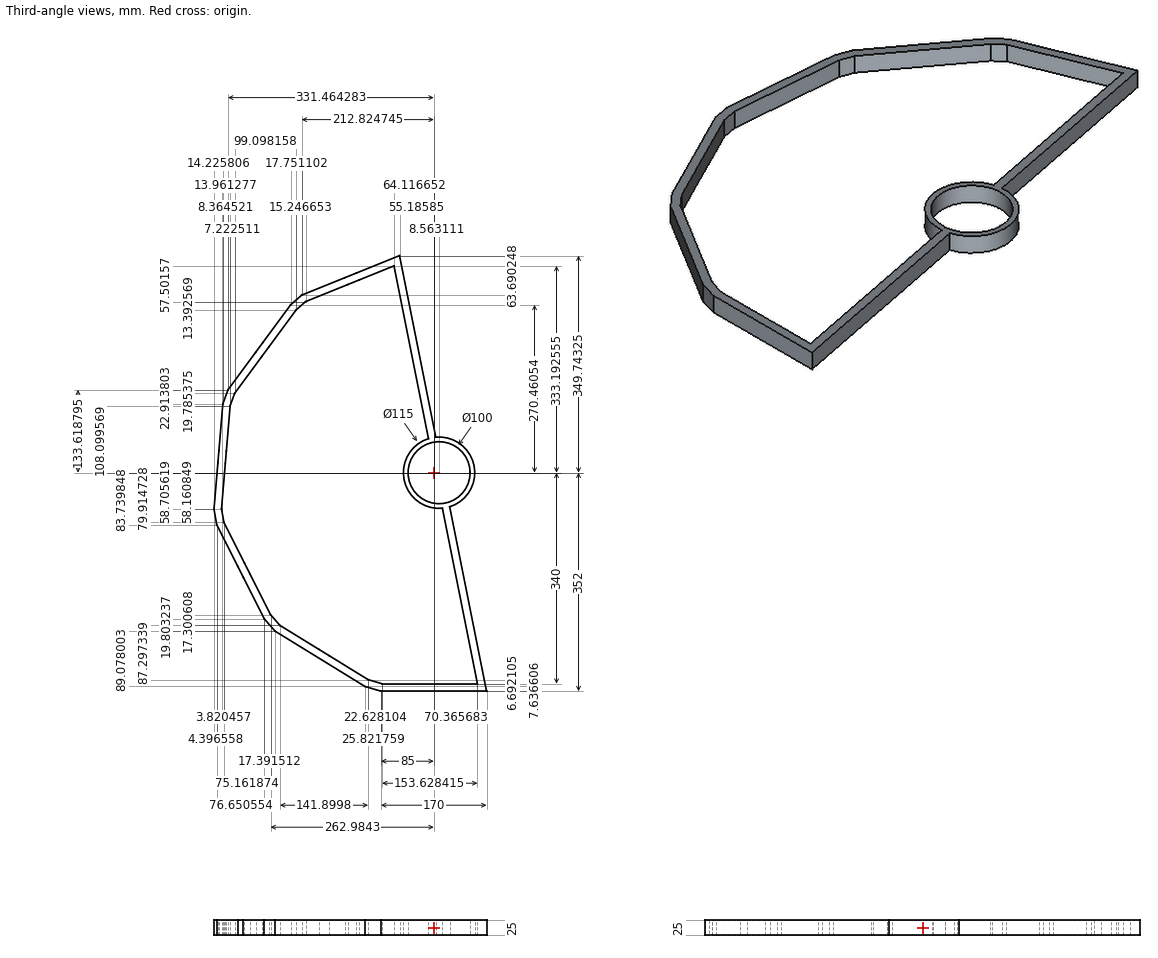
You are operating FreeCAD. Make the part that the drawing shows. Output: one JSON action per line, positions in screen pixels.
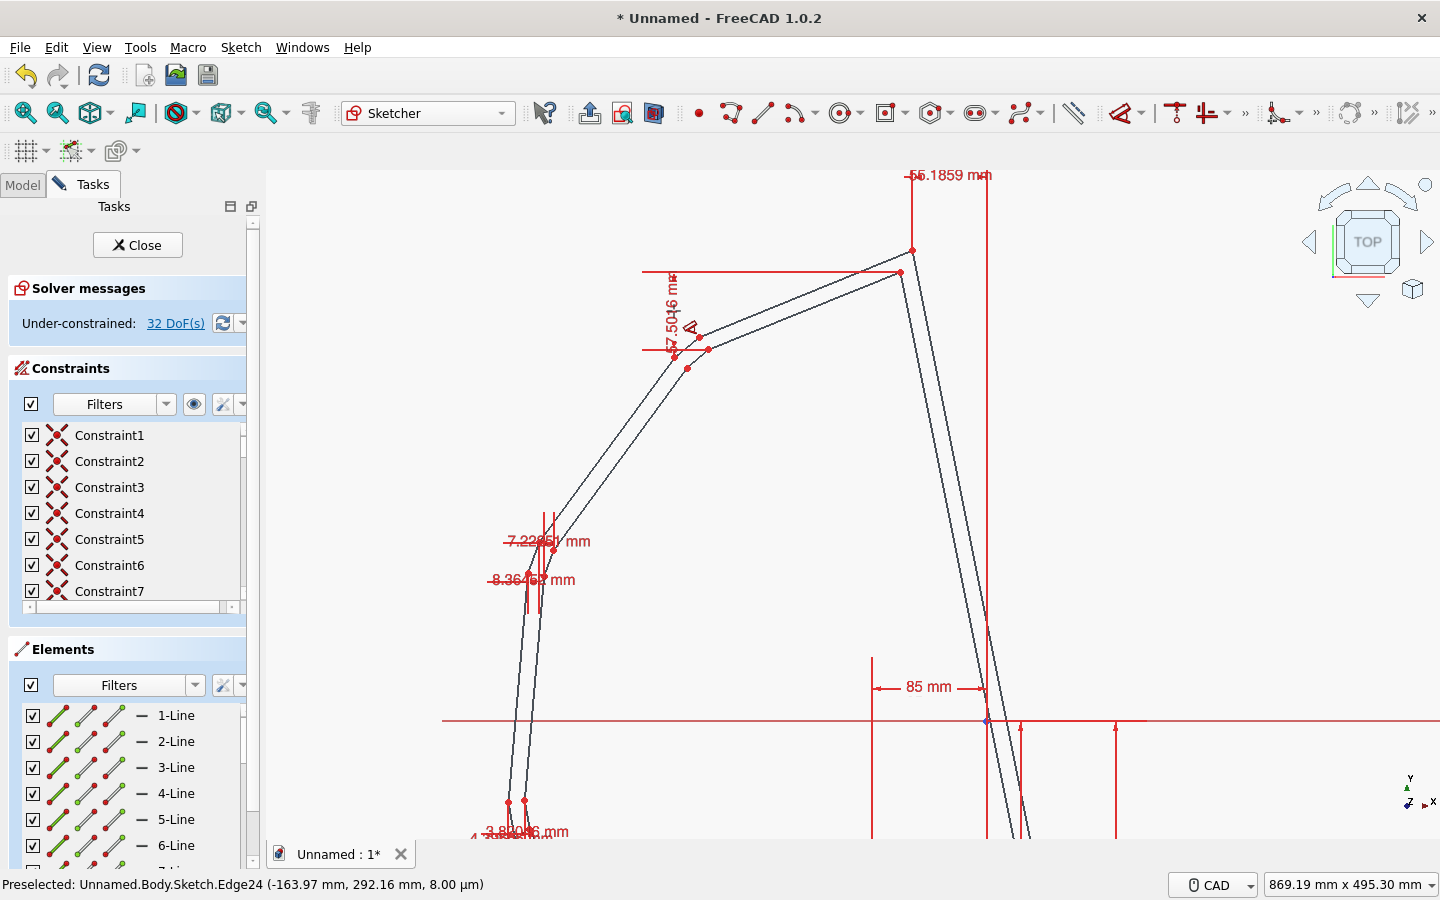
{"action": "scroll", "coordinate": [768, 326], "scroll_direction": "down", "scroll_amount": 4}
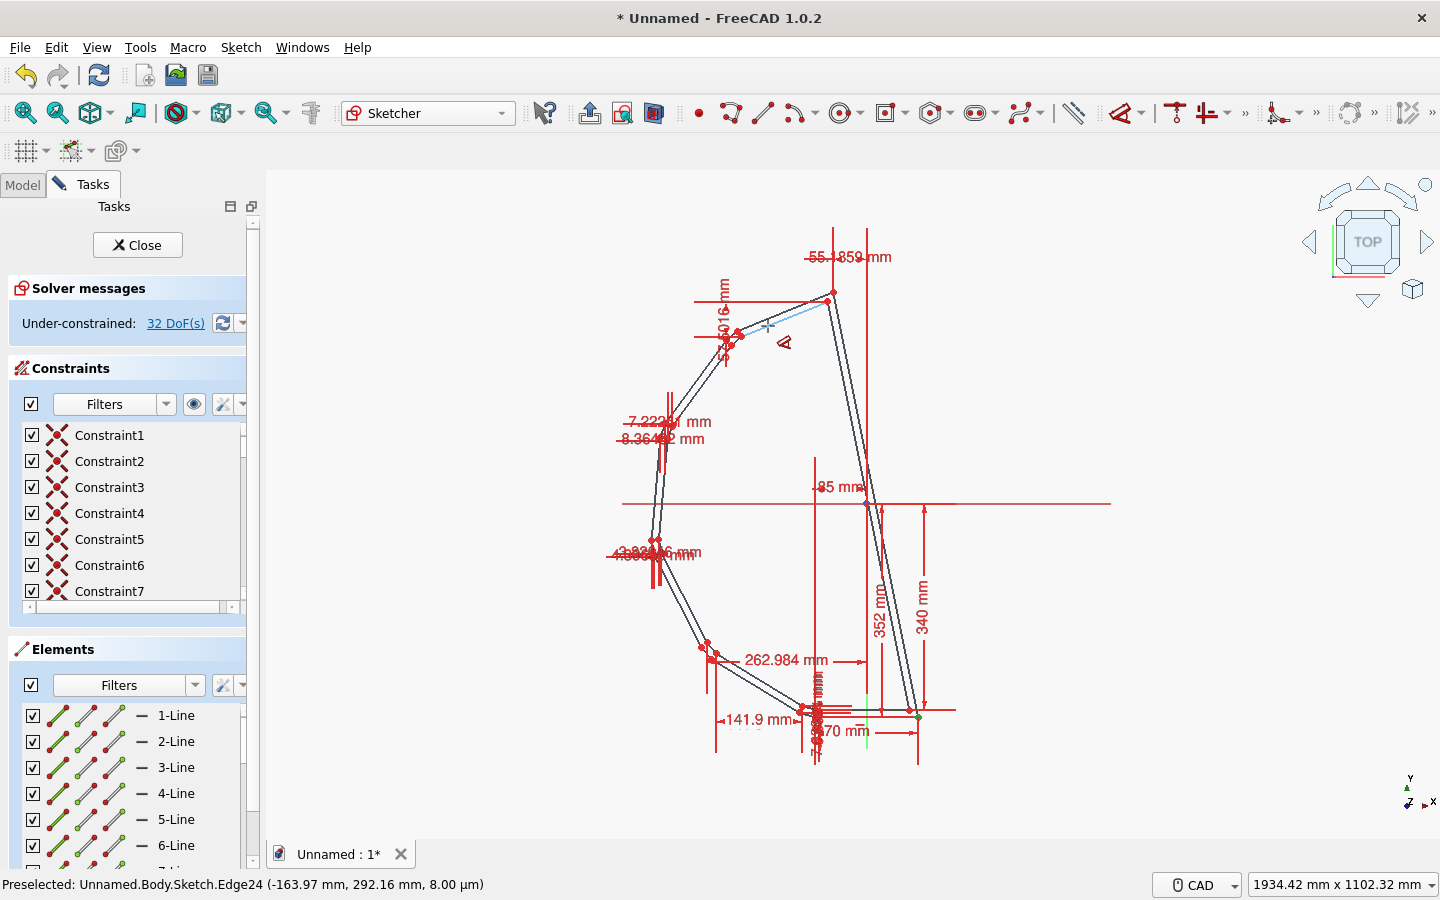
{"action": "scroll", "coordinate": [881, 710], "scroll_direction": "up", "scroll_amount": 4}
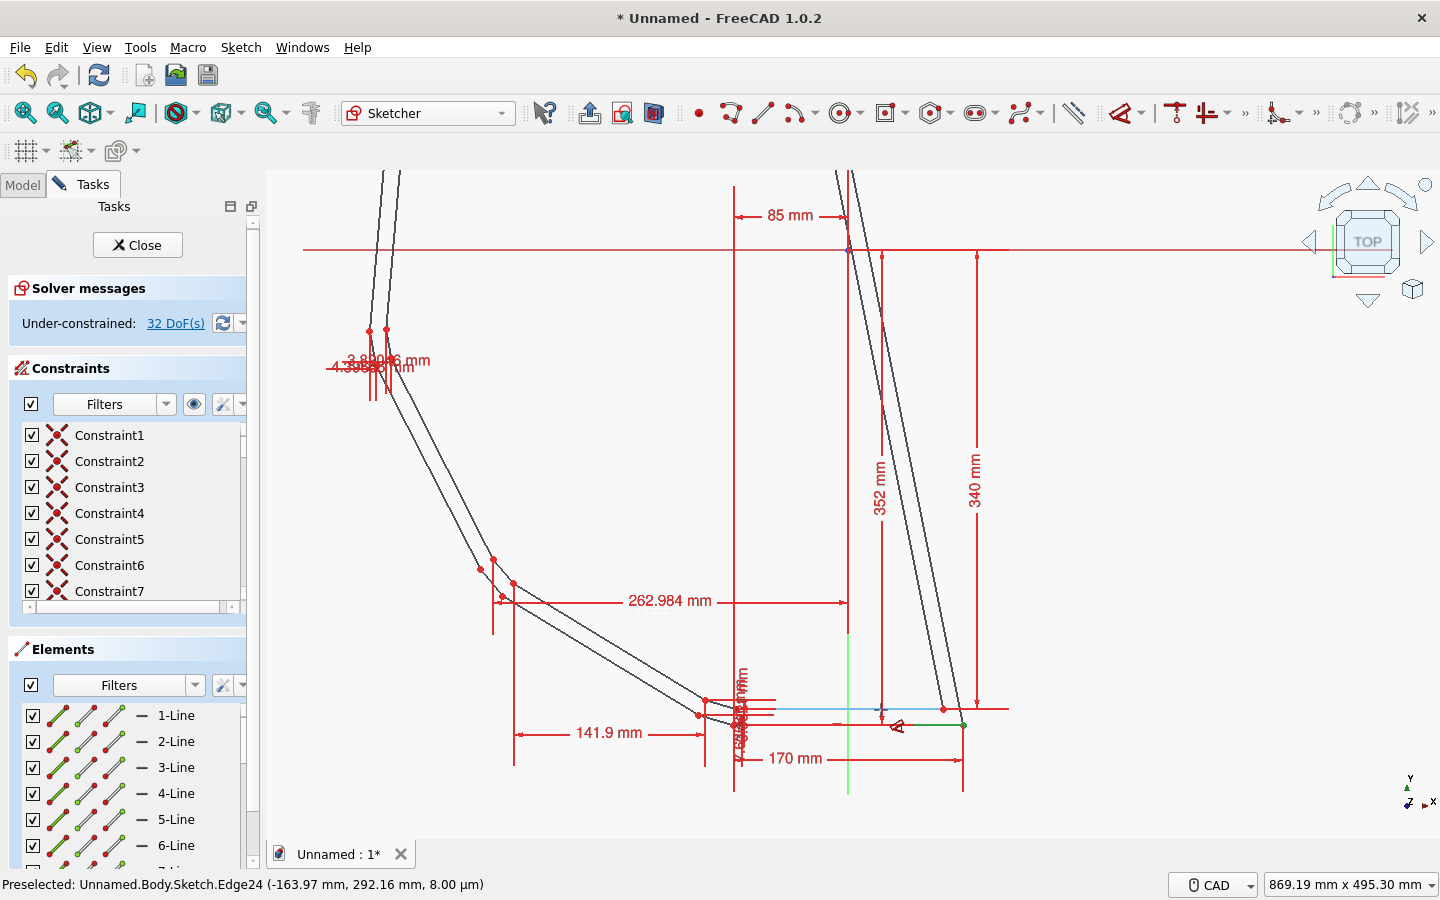
{"action": "left_click", "coordinate": [881, 709]}
{"action": "left_click", "coordinate": [887, 743]}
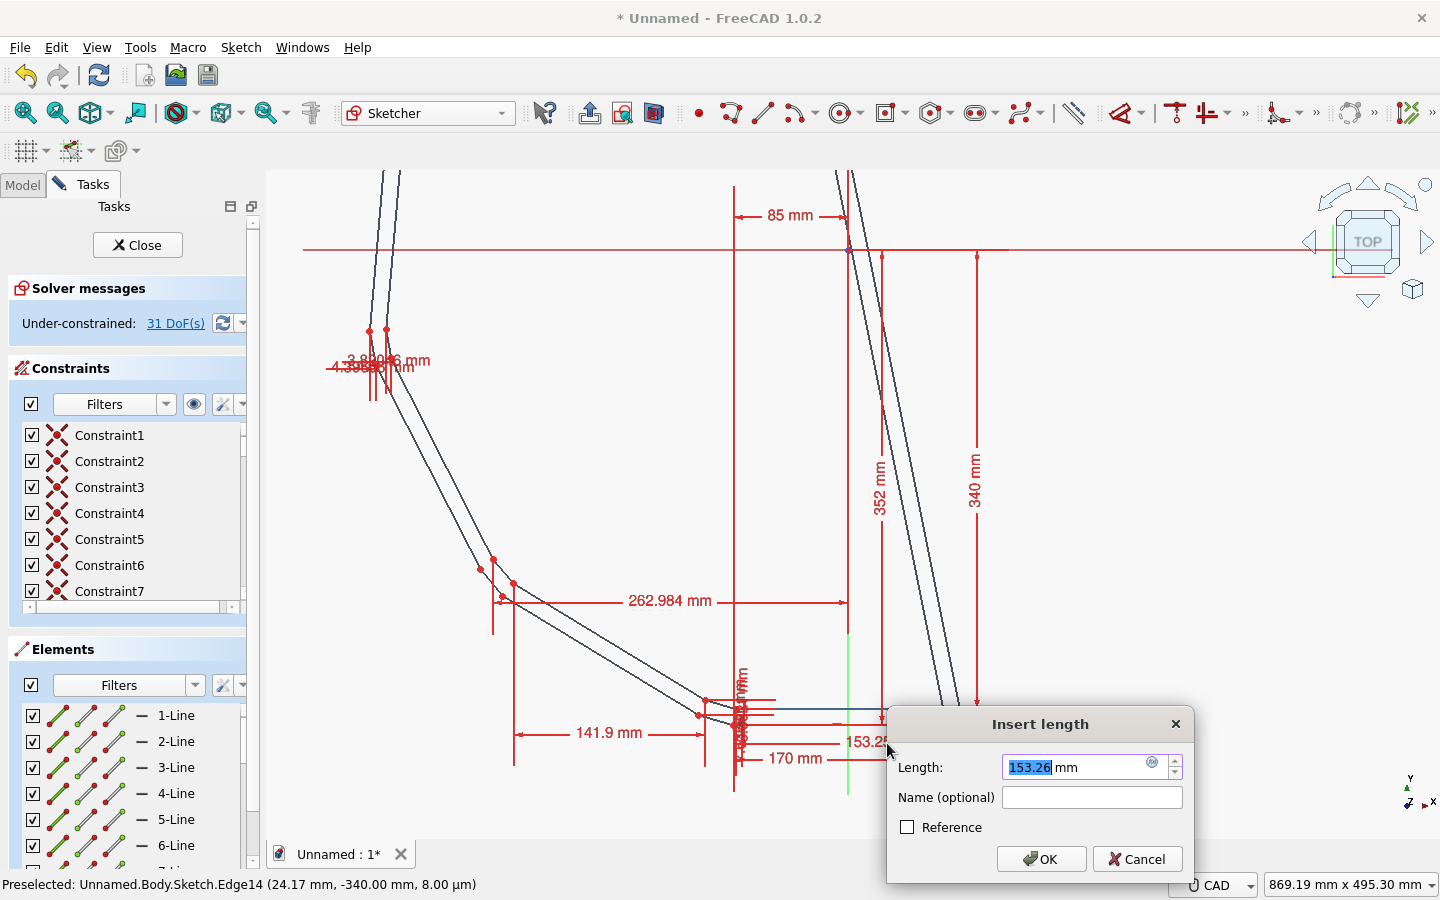
{"action": "type", "text": "153.628415"}
{"action": "key", "text": "Return"}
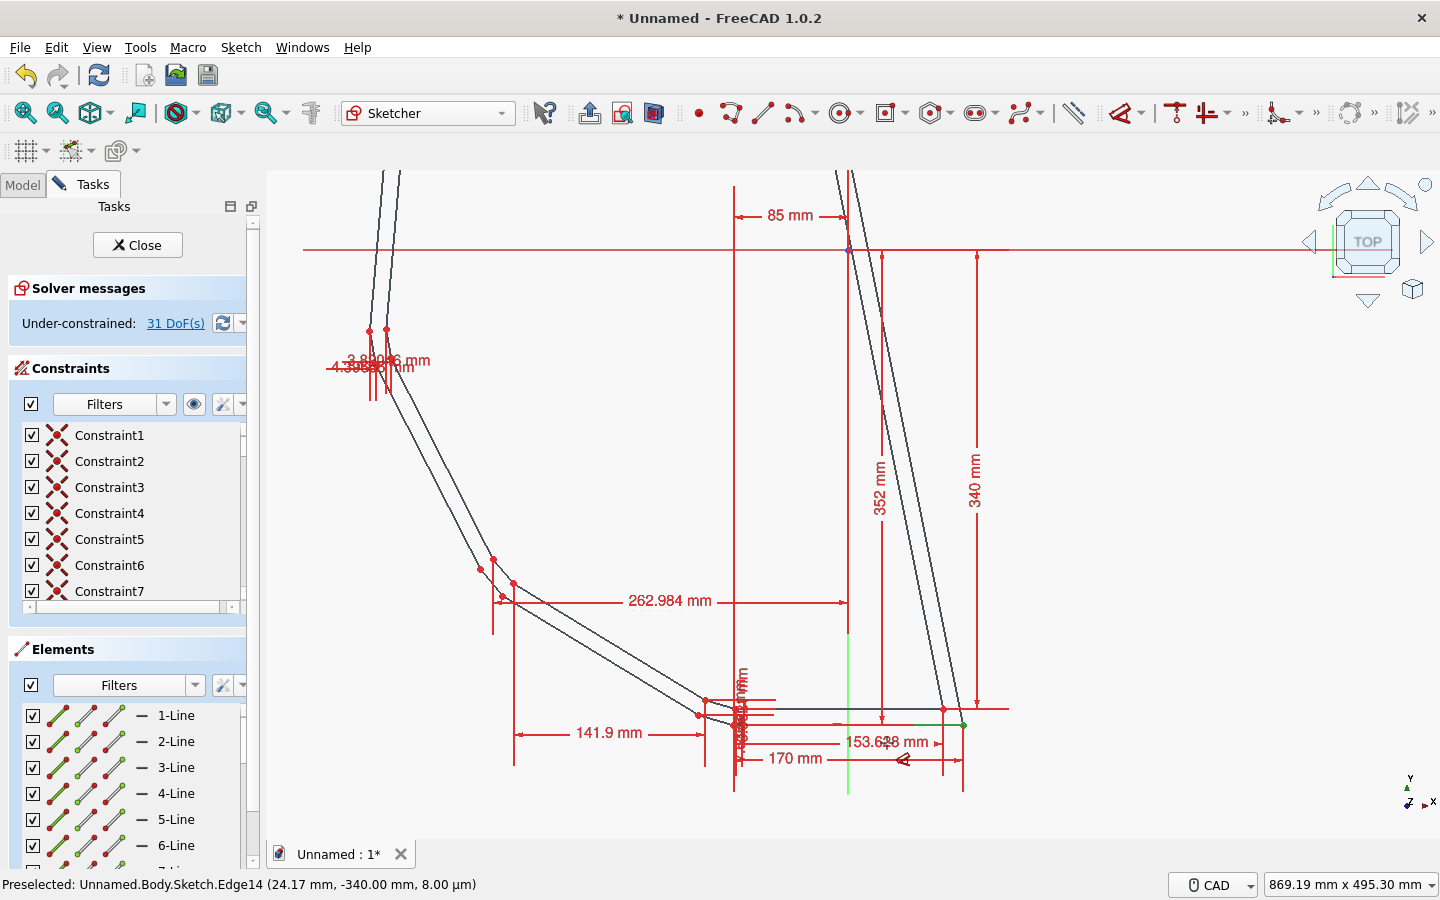
{"action": "scroll", "coordinate": [881, 711], "scroll_direction": "down", "scroll_amount": 4}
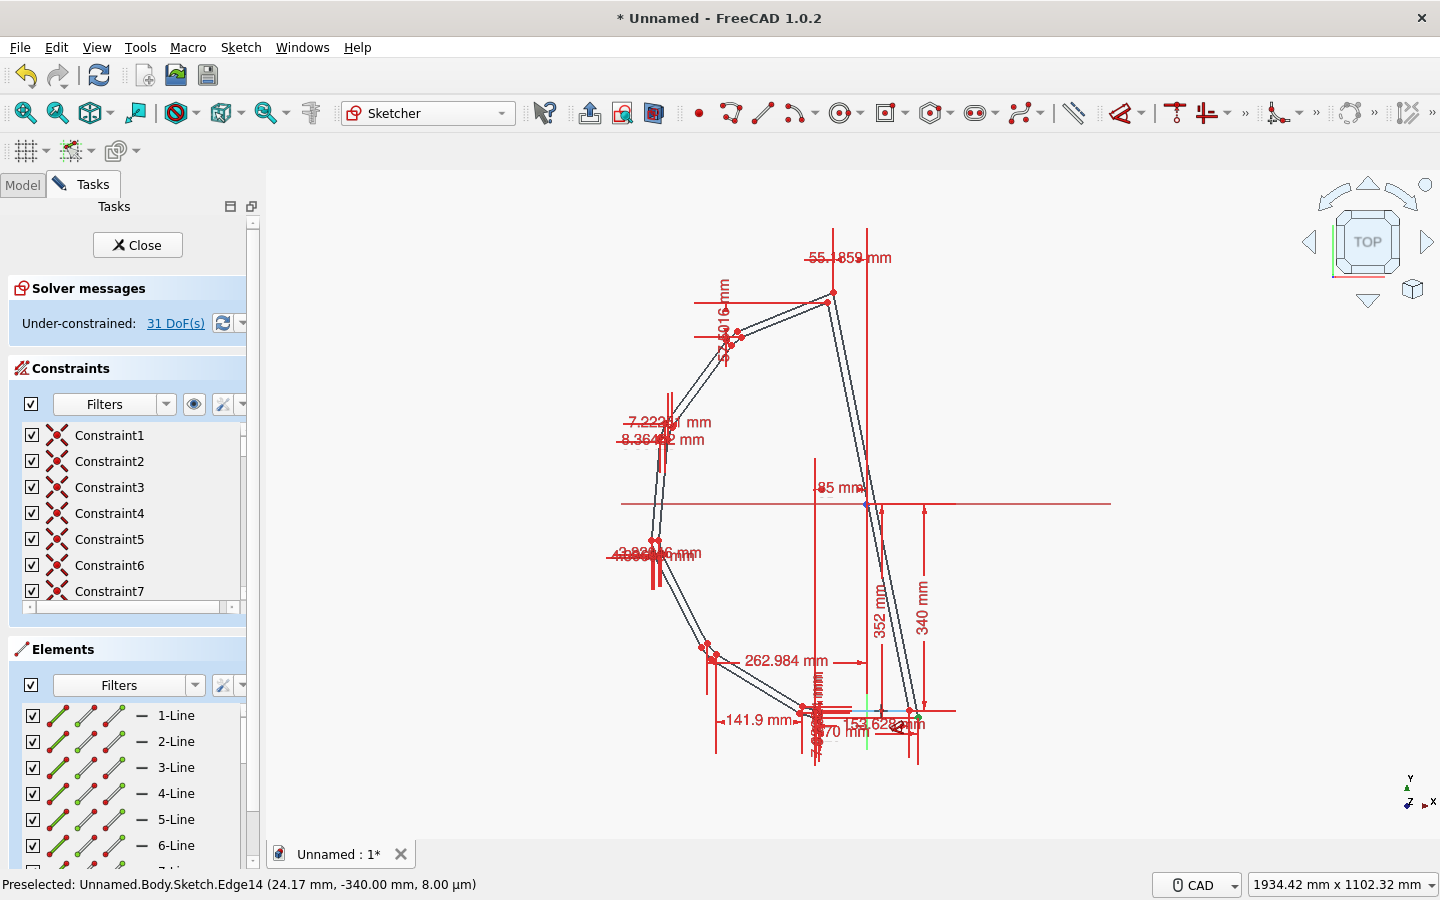
{"action": "left_click", "coordinate": [833, 293]}
{"action": "left_click", "coordinate": [901, 399]}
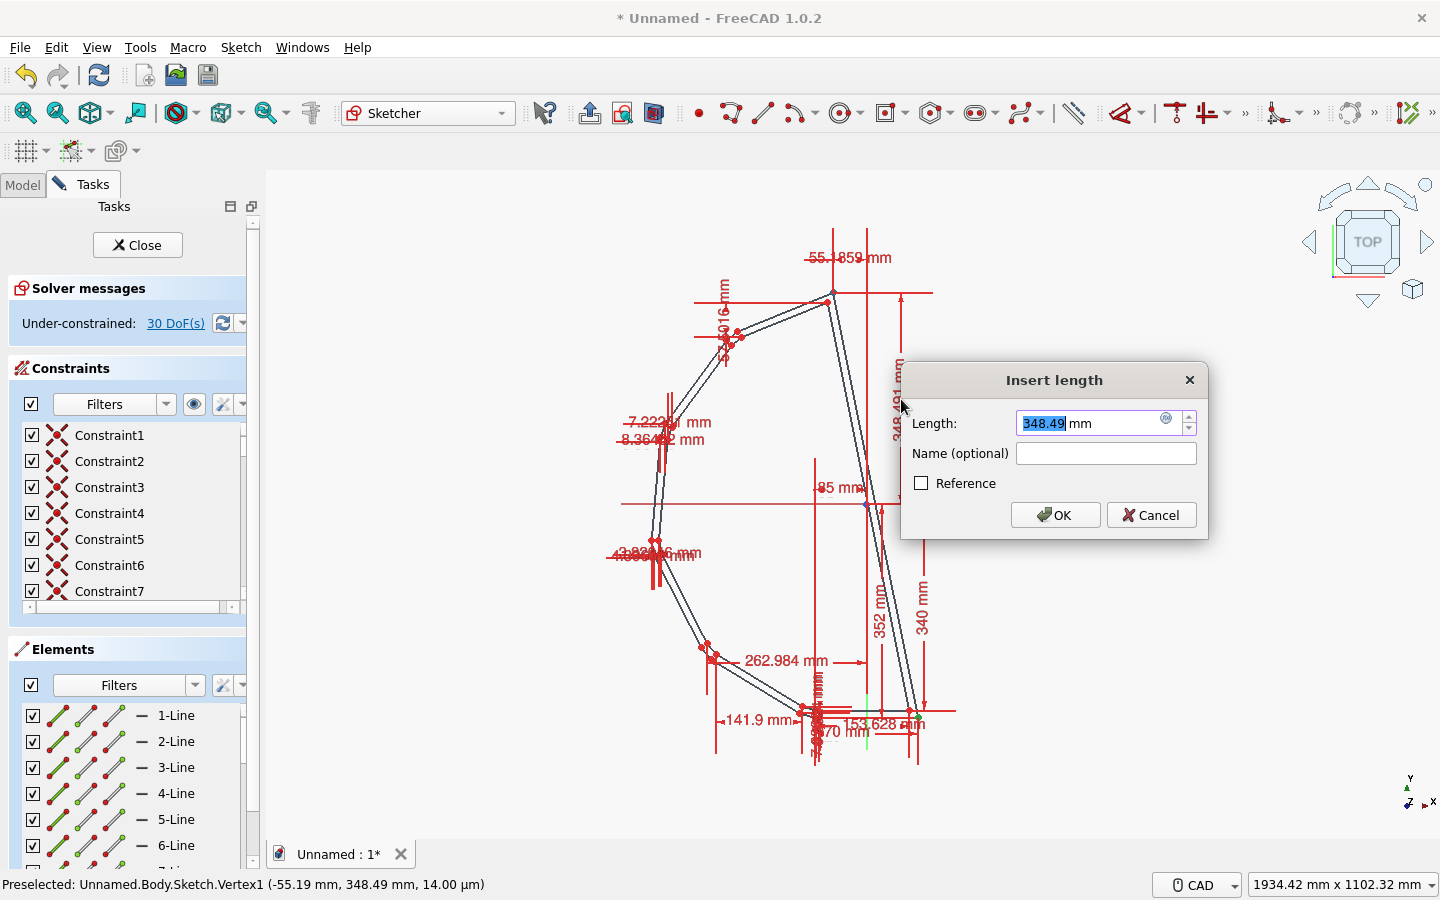
{"action": "type", "text": "349.74325"}
{"action": "key", "text": "Return"}